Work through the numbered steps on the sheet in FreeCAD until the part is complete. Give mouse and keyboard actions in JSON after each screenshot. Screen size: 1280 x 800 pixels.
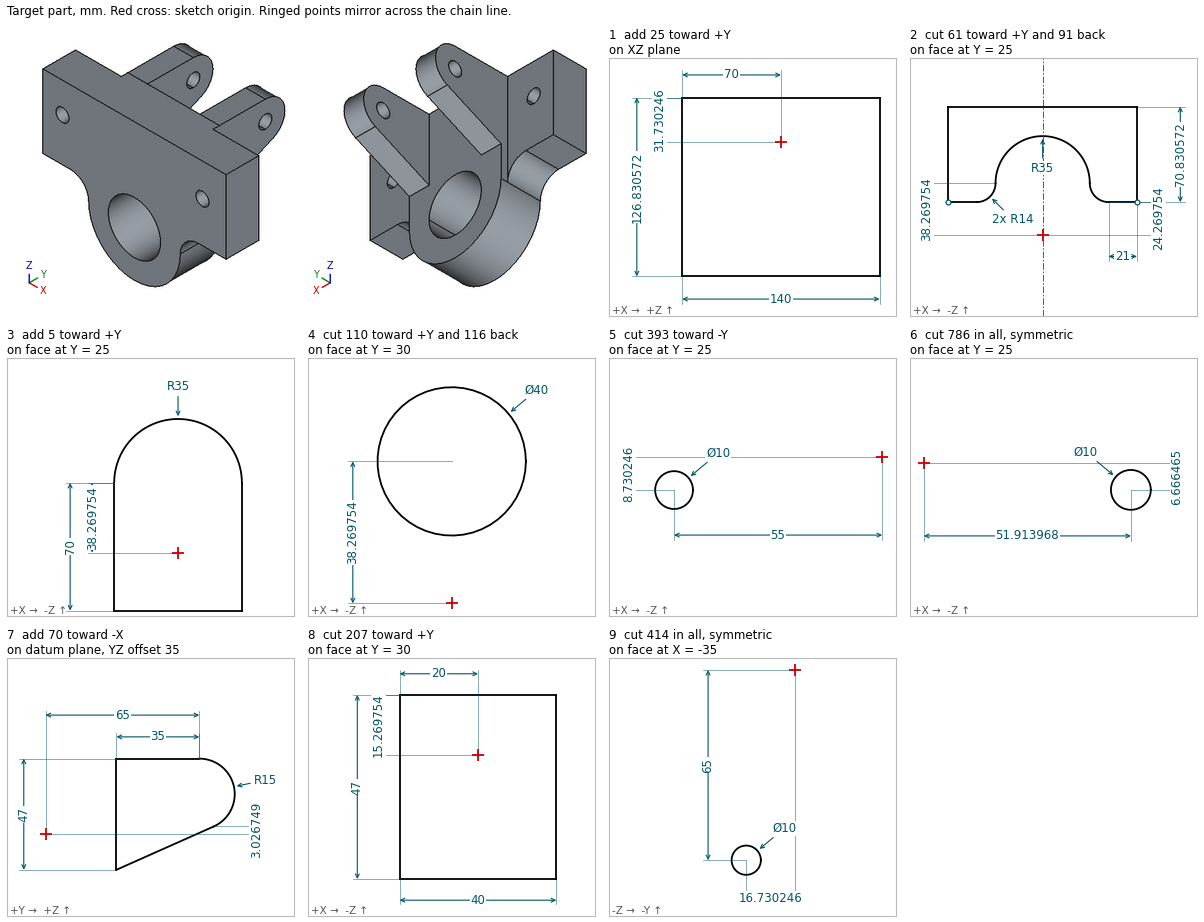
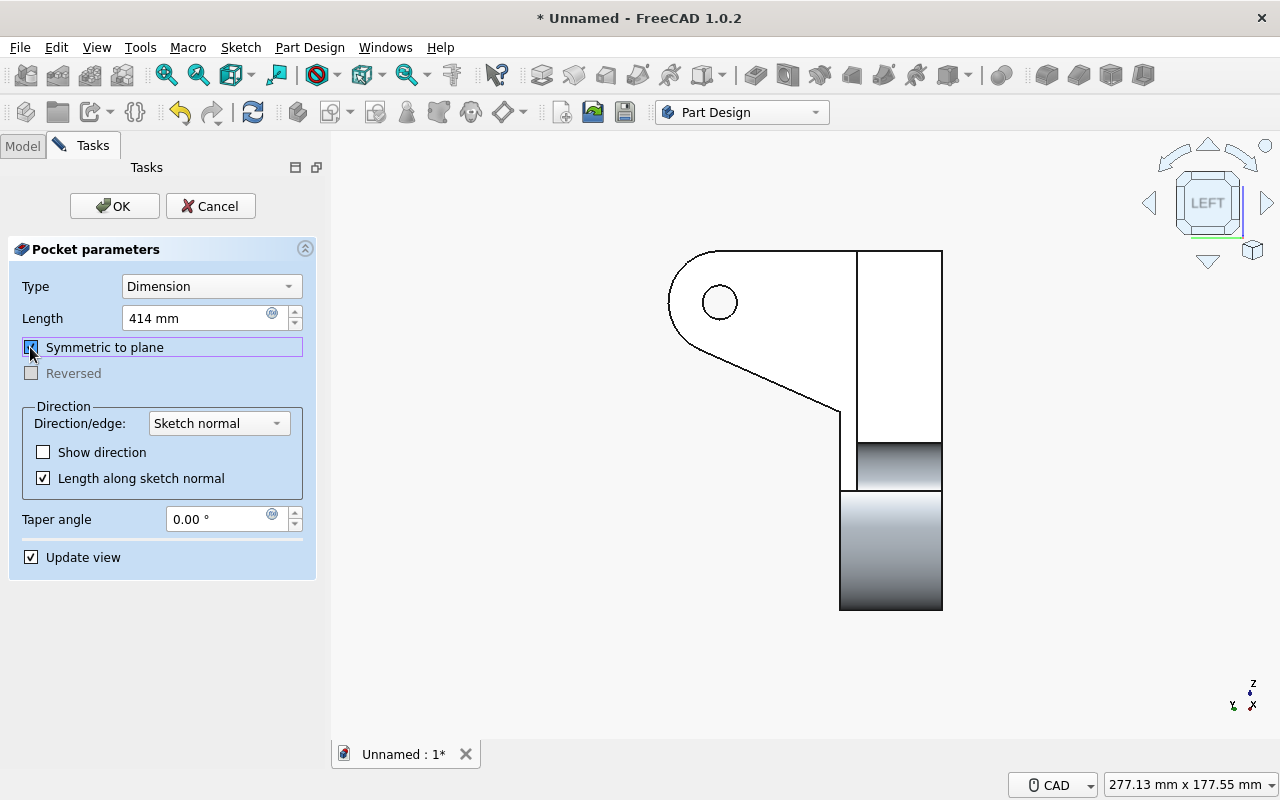
{"action": "left_click", "coordinate": [115, 206]}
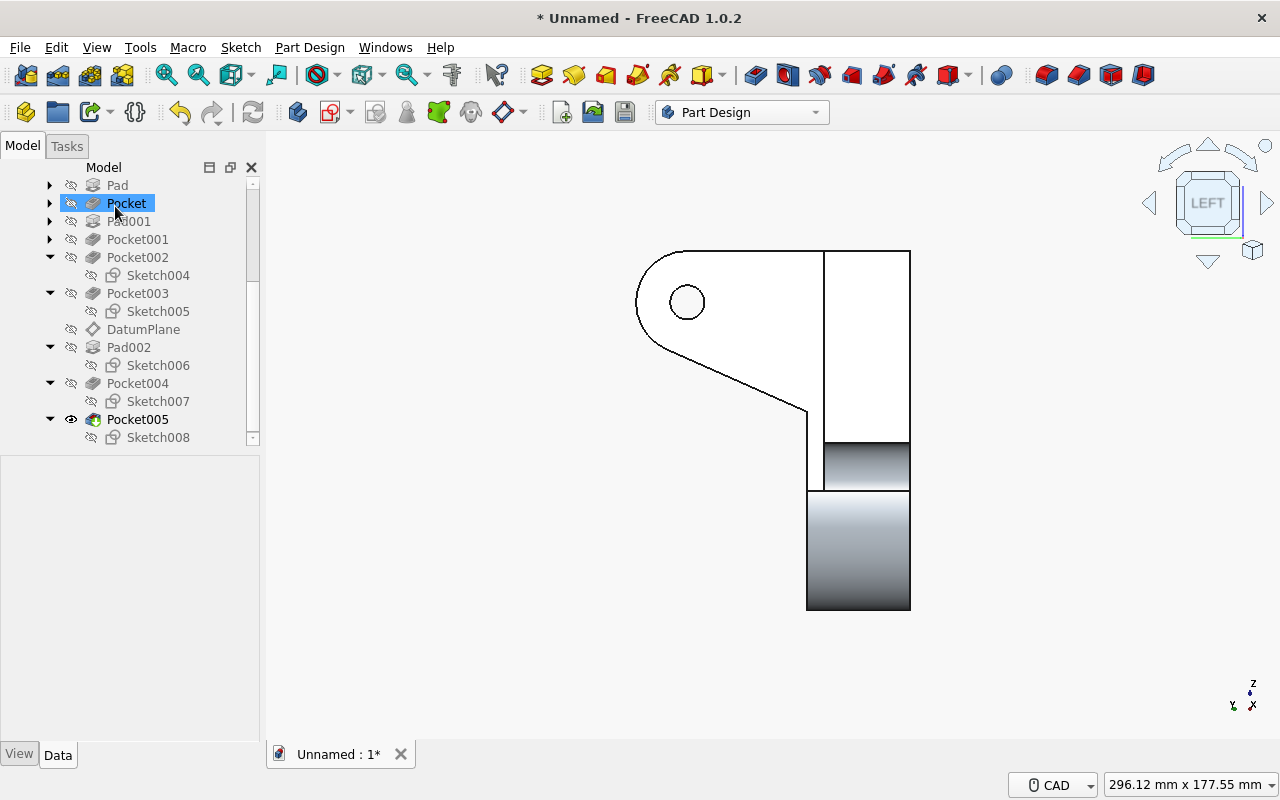
{"action": "key", "text": "0"}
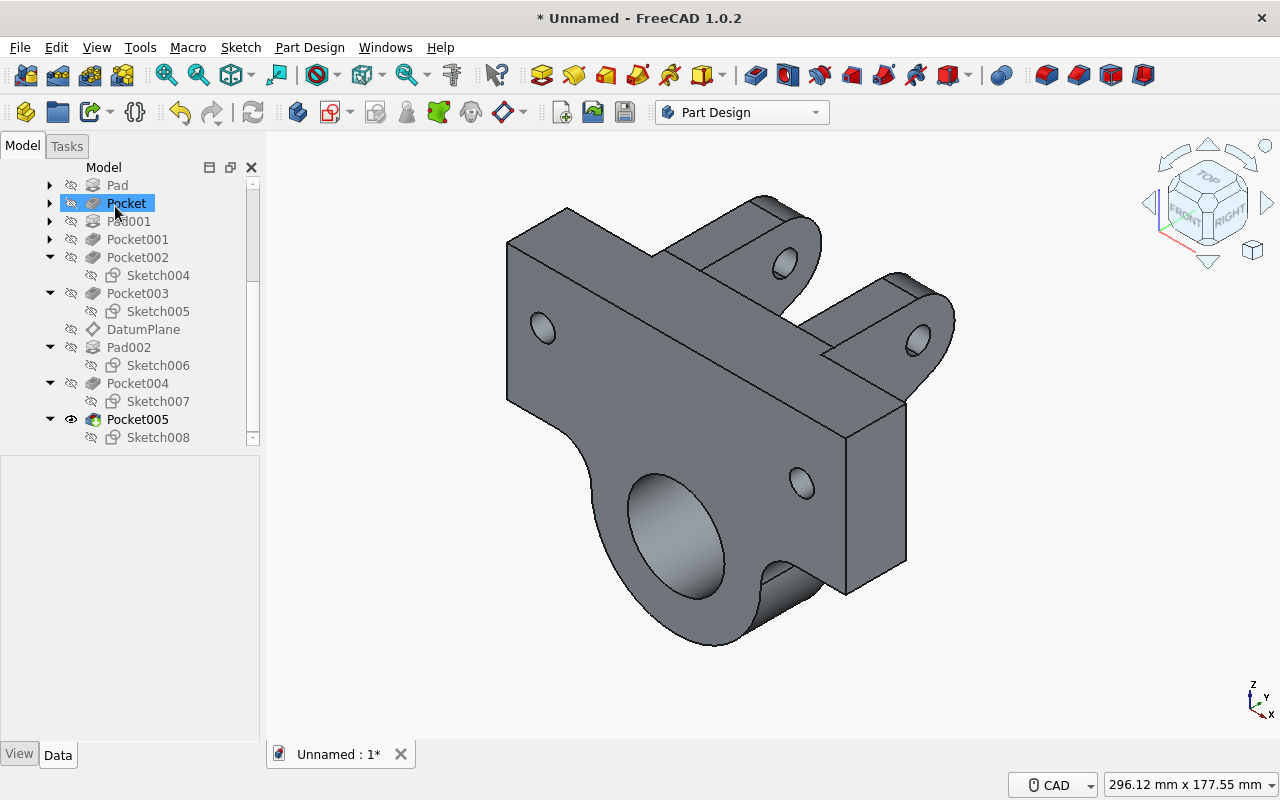
{"action": "left_click", "coordinate": [168, 76]}